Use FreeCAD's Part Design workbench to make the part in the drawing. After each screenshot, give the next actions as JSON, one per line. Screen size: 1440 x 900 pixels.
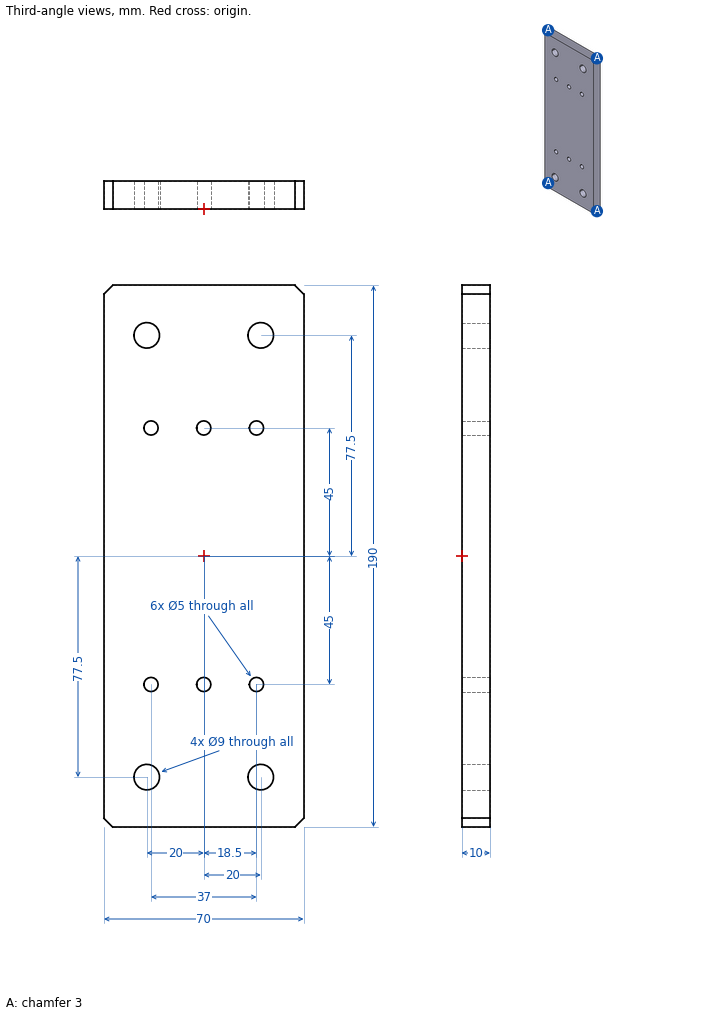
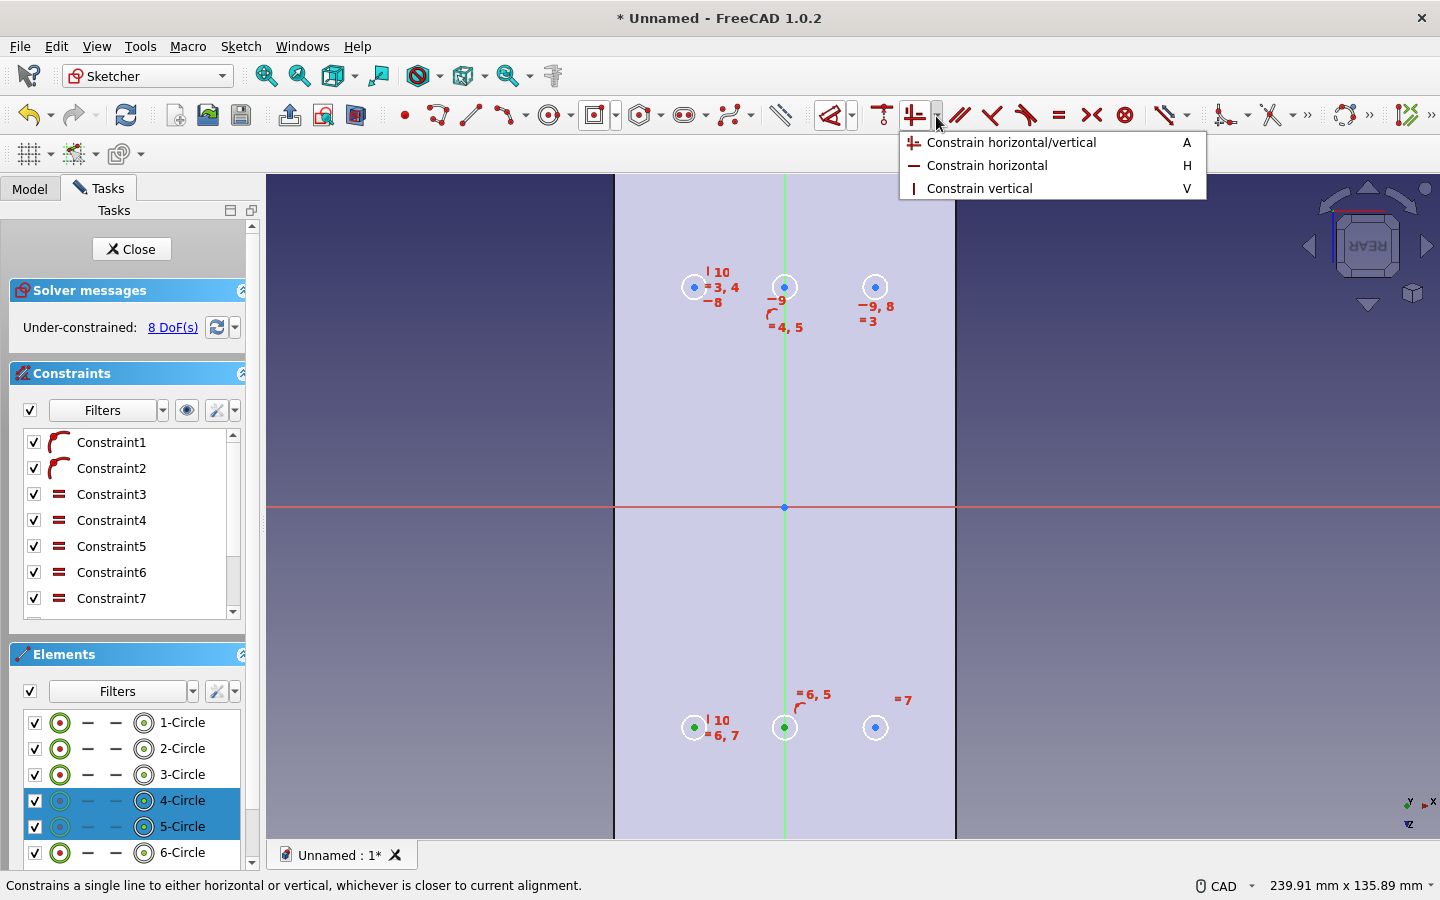
{"action": "left_click", "coordinate": [1053, 166]}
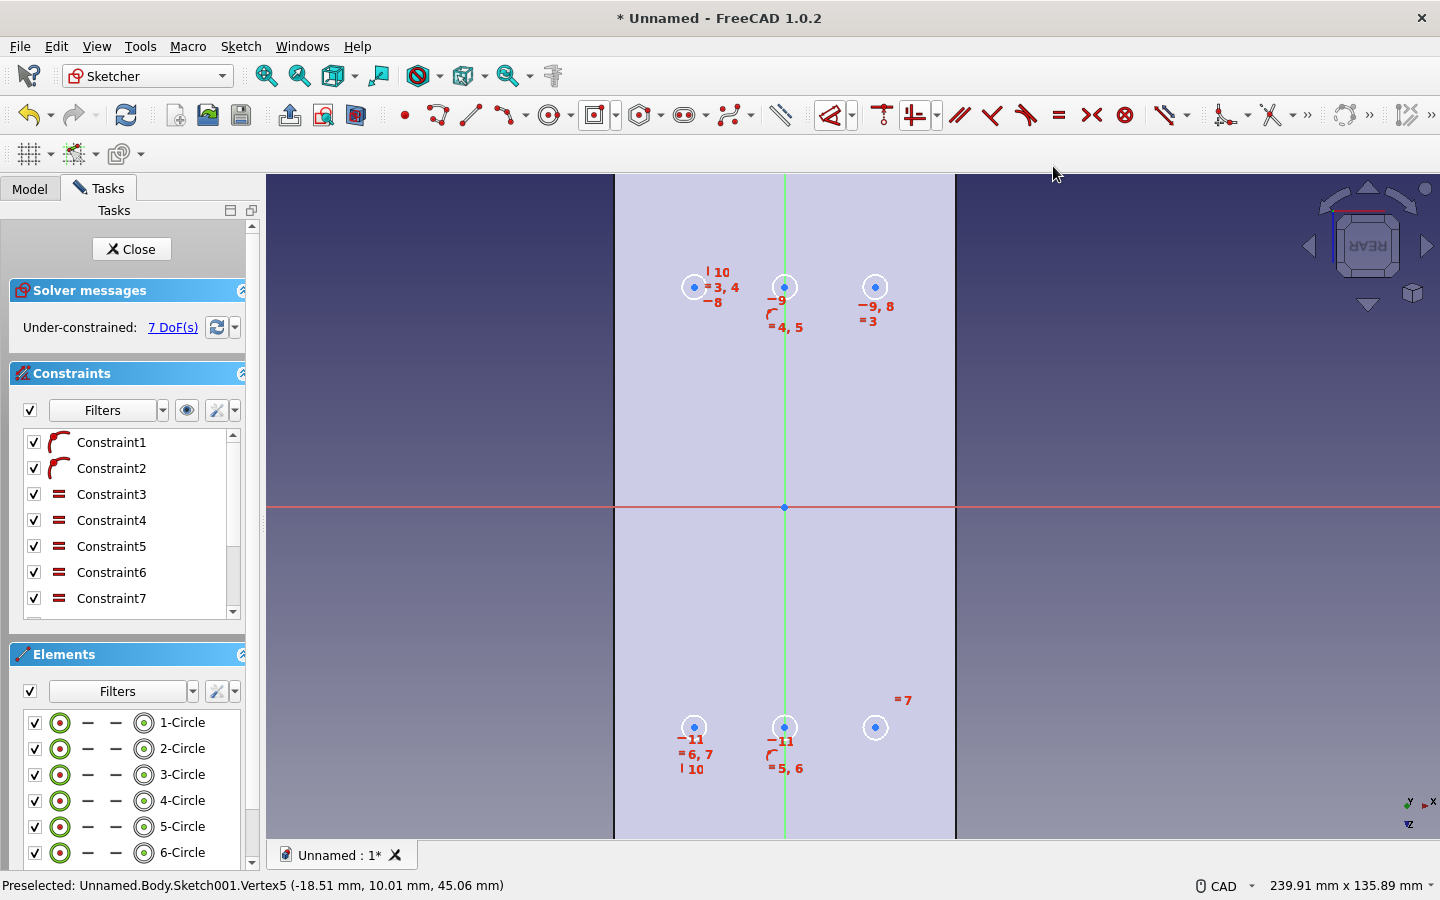
{"action": "left_click", "coordinate": [875, 287]}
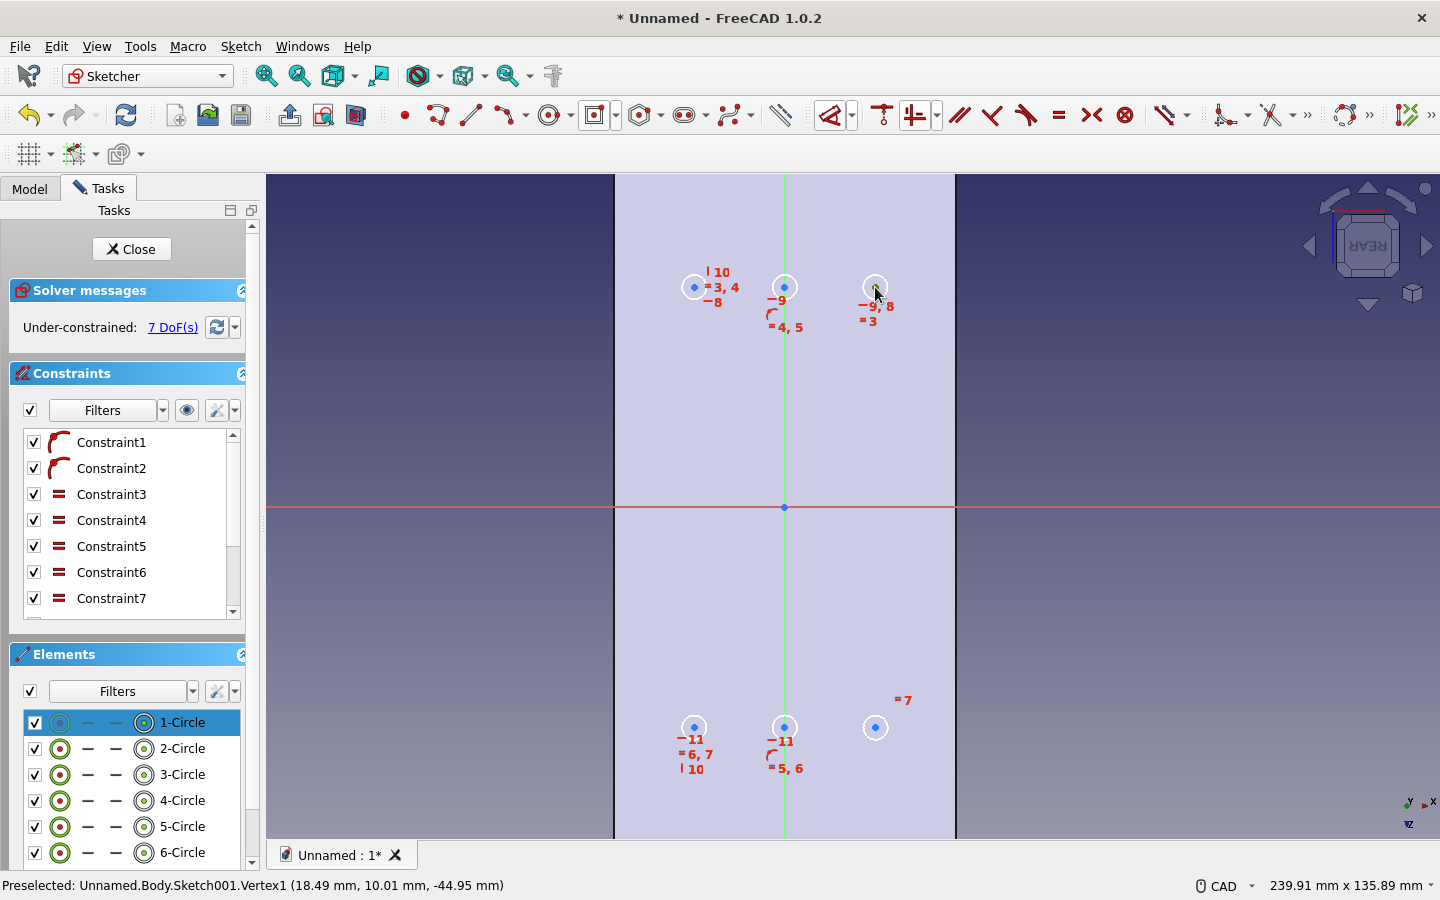
{"action": "left_click", "coordinate": [876, 728]}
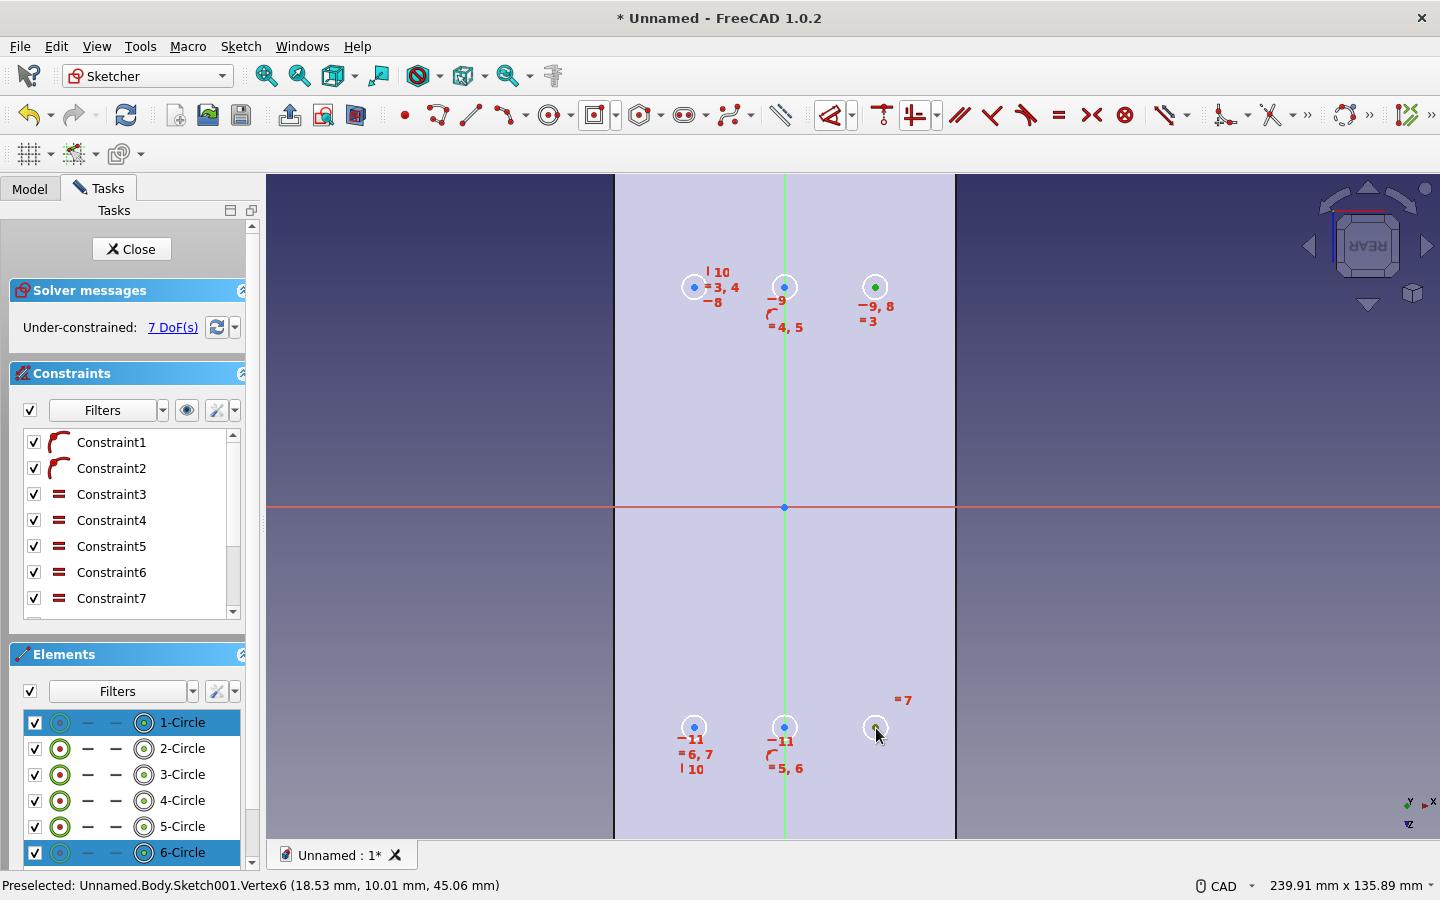
{"action": "key", "text": "v"}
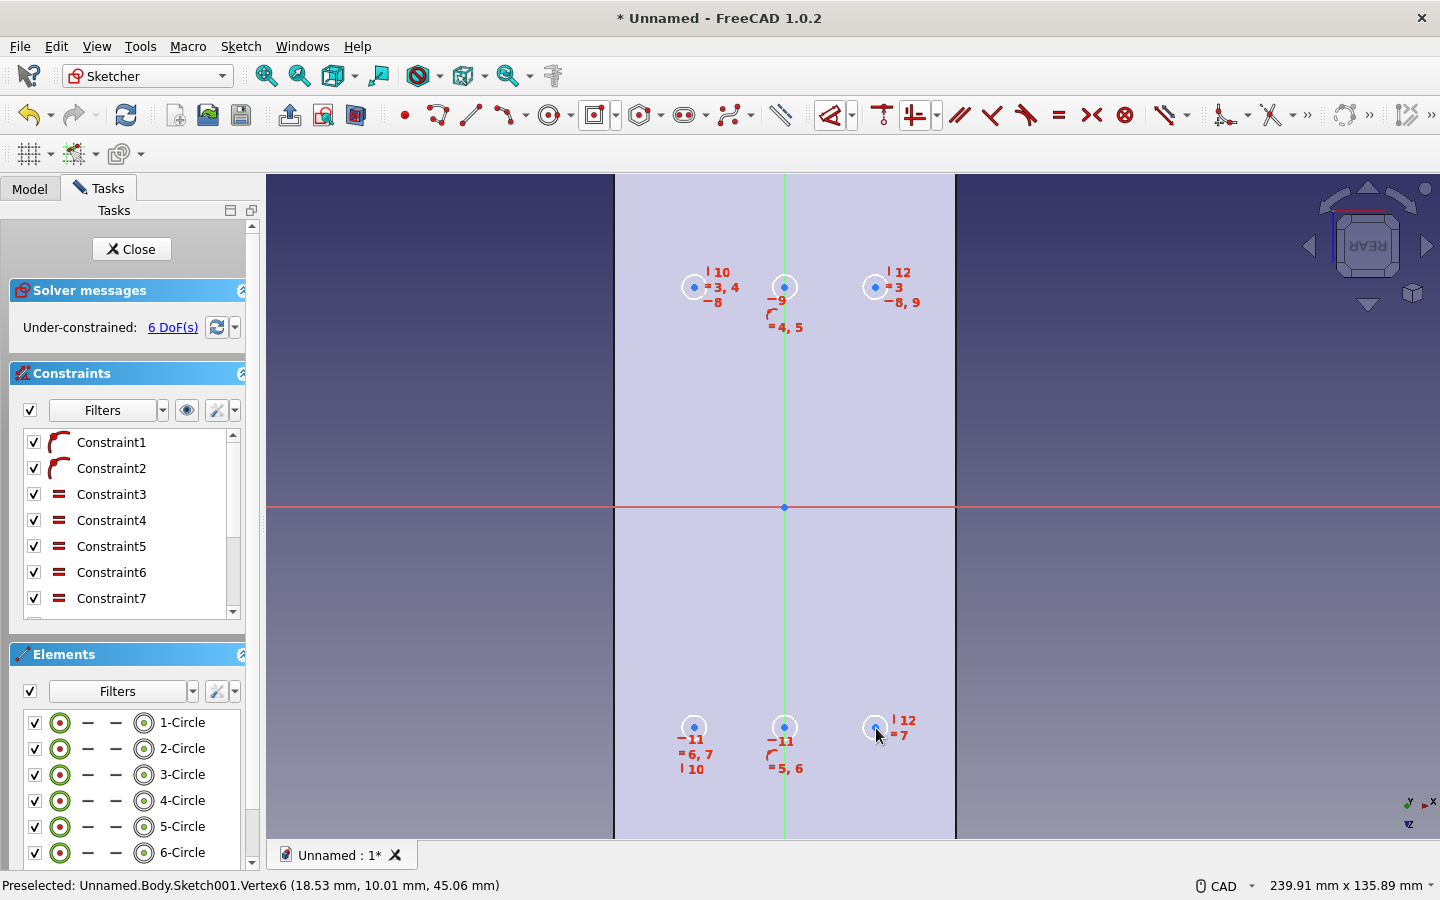
{"action": "left_click", "coordinate": [785, 728]}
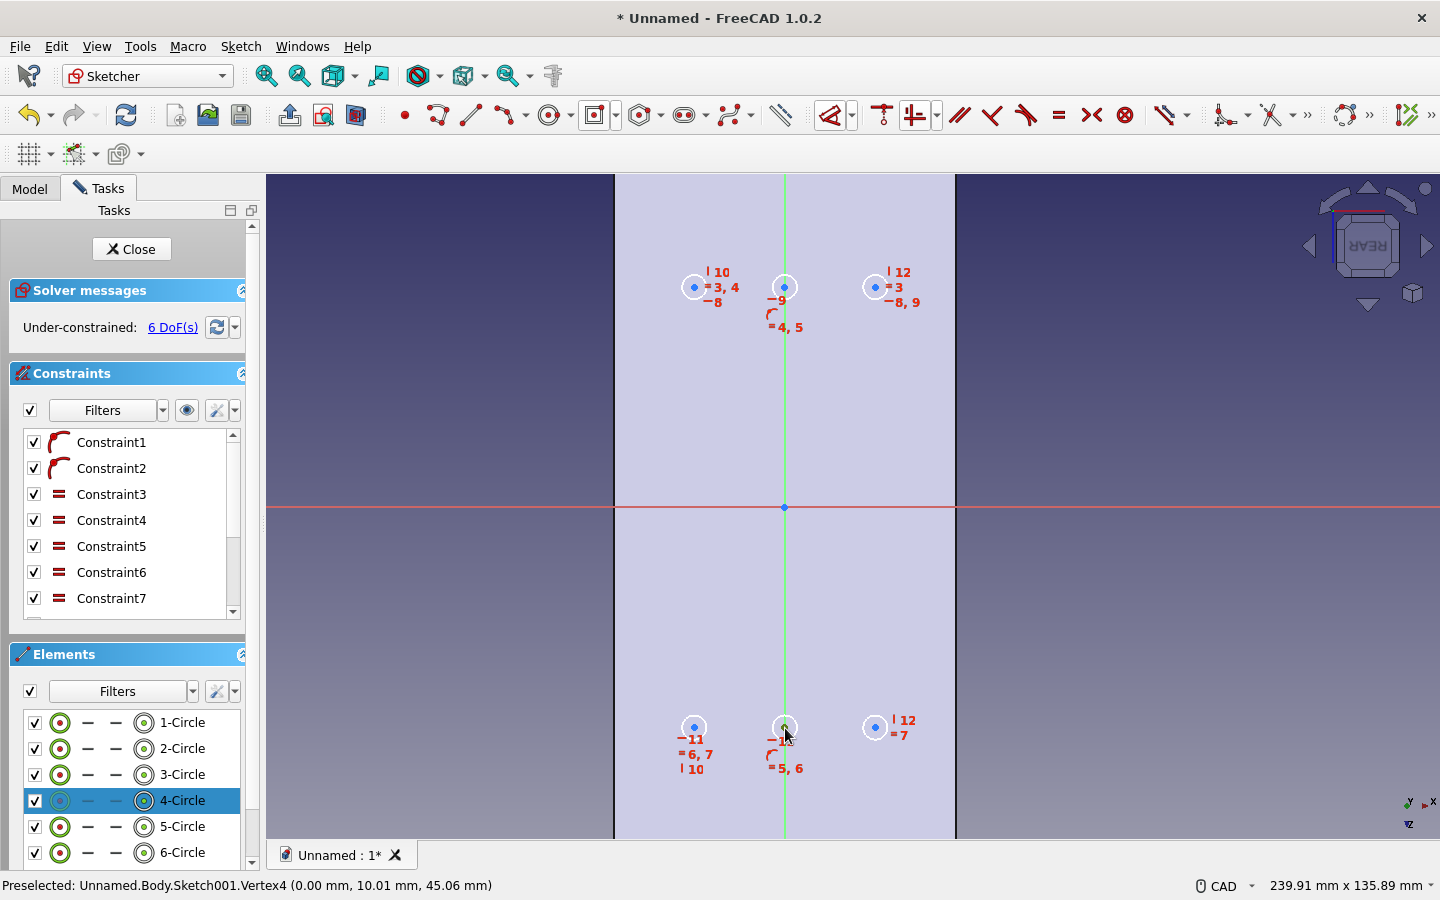
{"action": "left_click", "coordinate": [875, 728]}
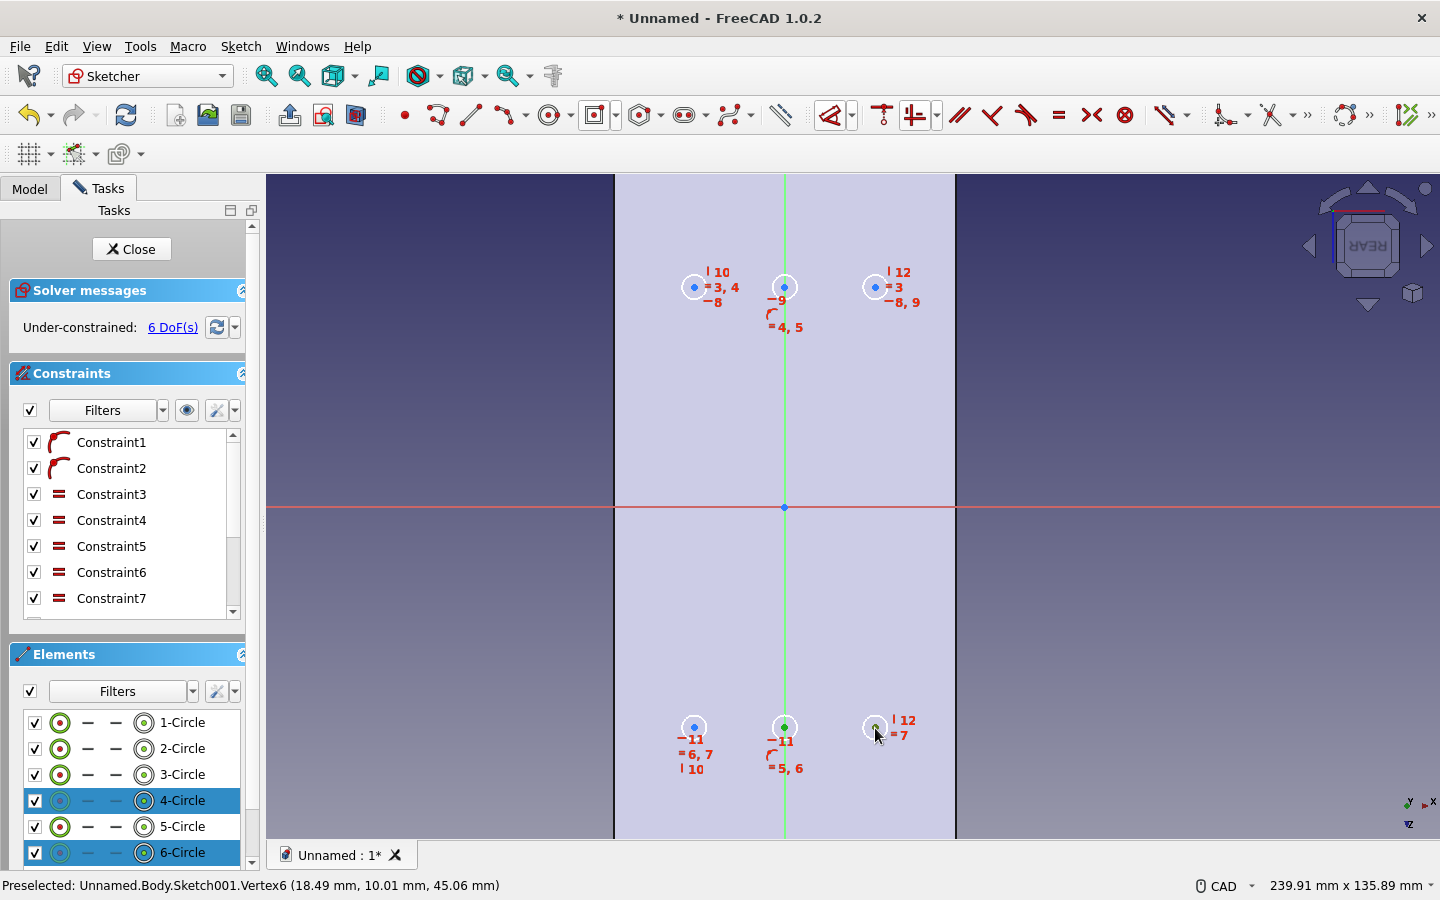
{"action": "left_click", "coordinate": [936, 116]}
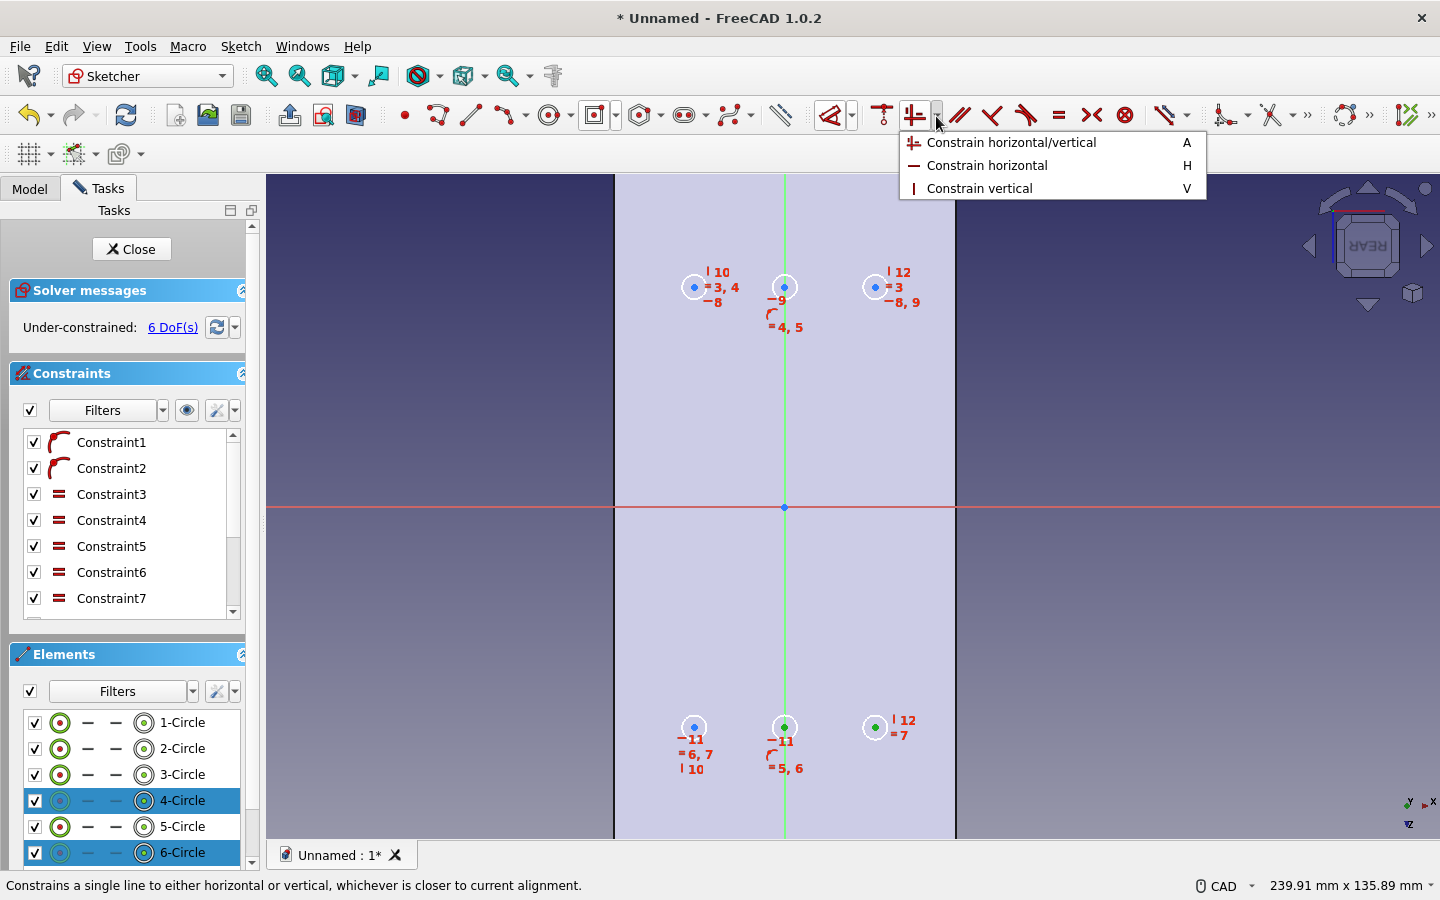
{"action": "left_click", "coordinate": [1053, 166]}